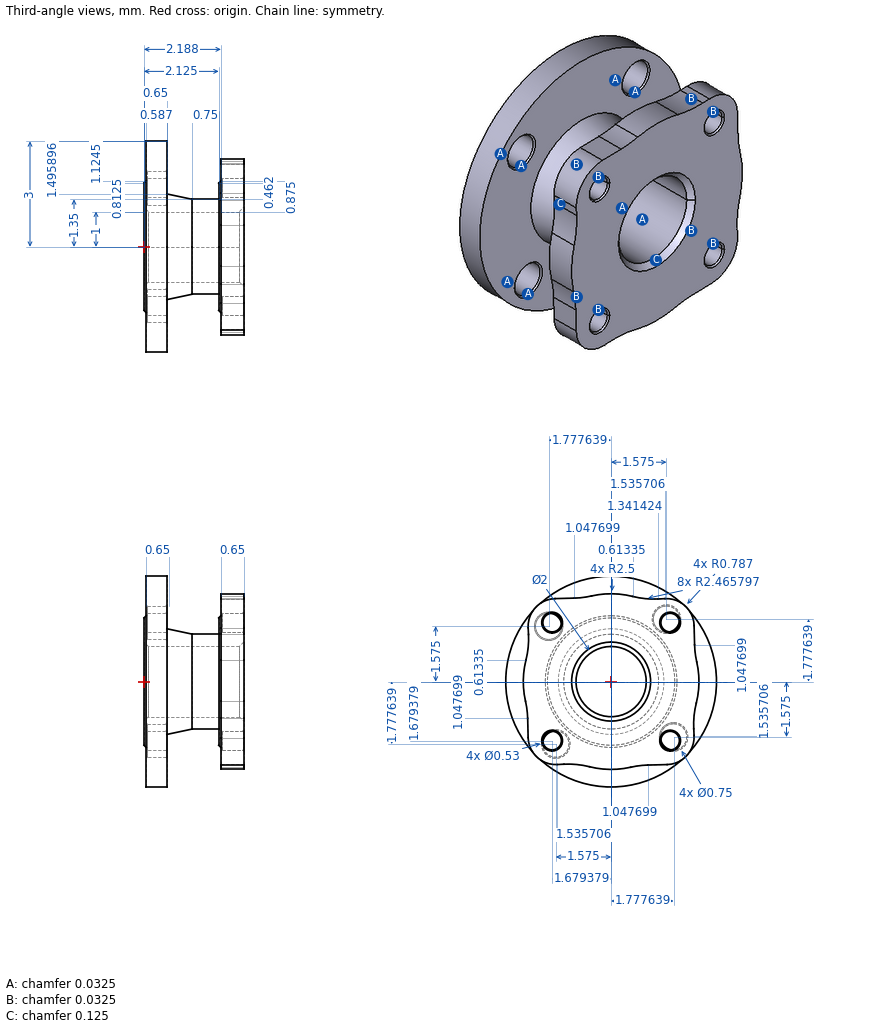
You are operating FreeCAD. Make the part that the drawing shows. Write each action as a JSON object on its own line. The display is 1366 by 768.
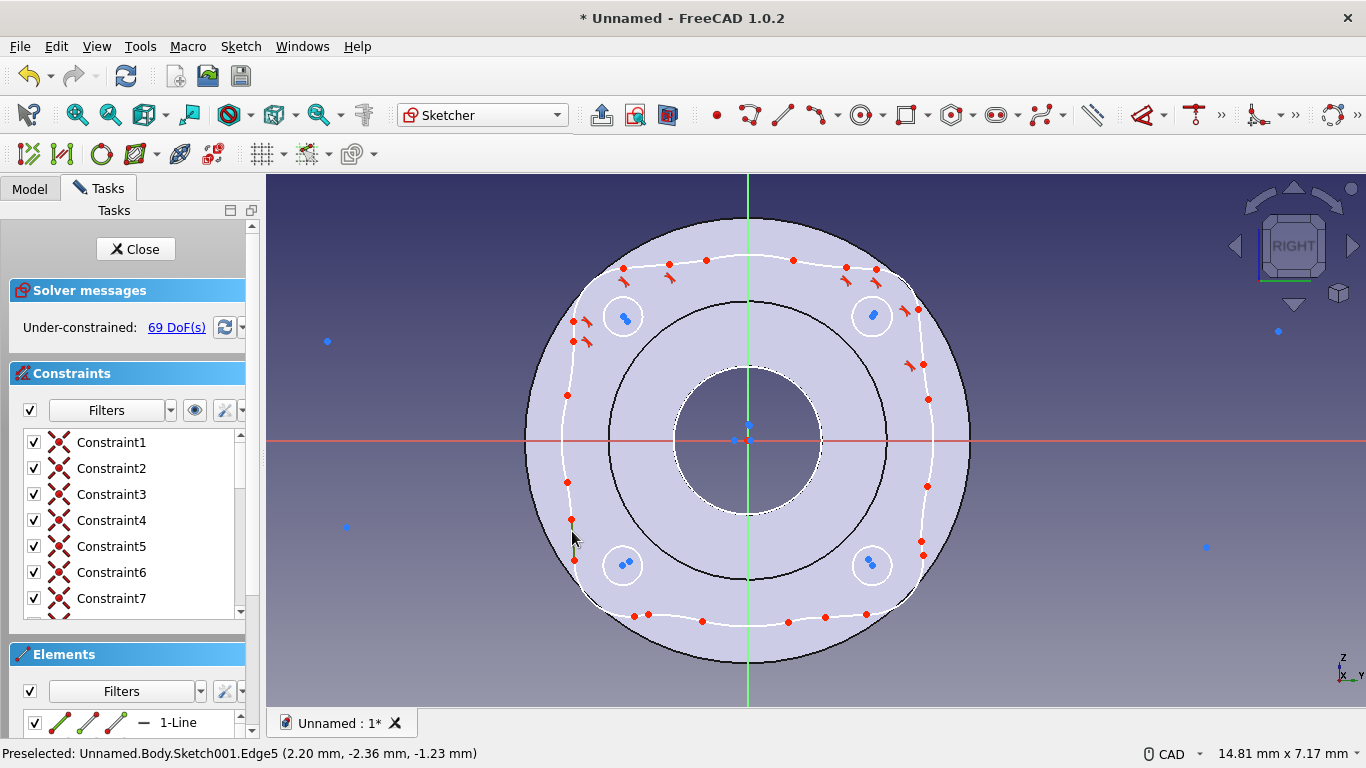
{"action": "scroll", "coordinate": [571, 508], "scroll_direction": "up", "scroll_amount": 2}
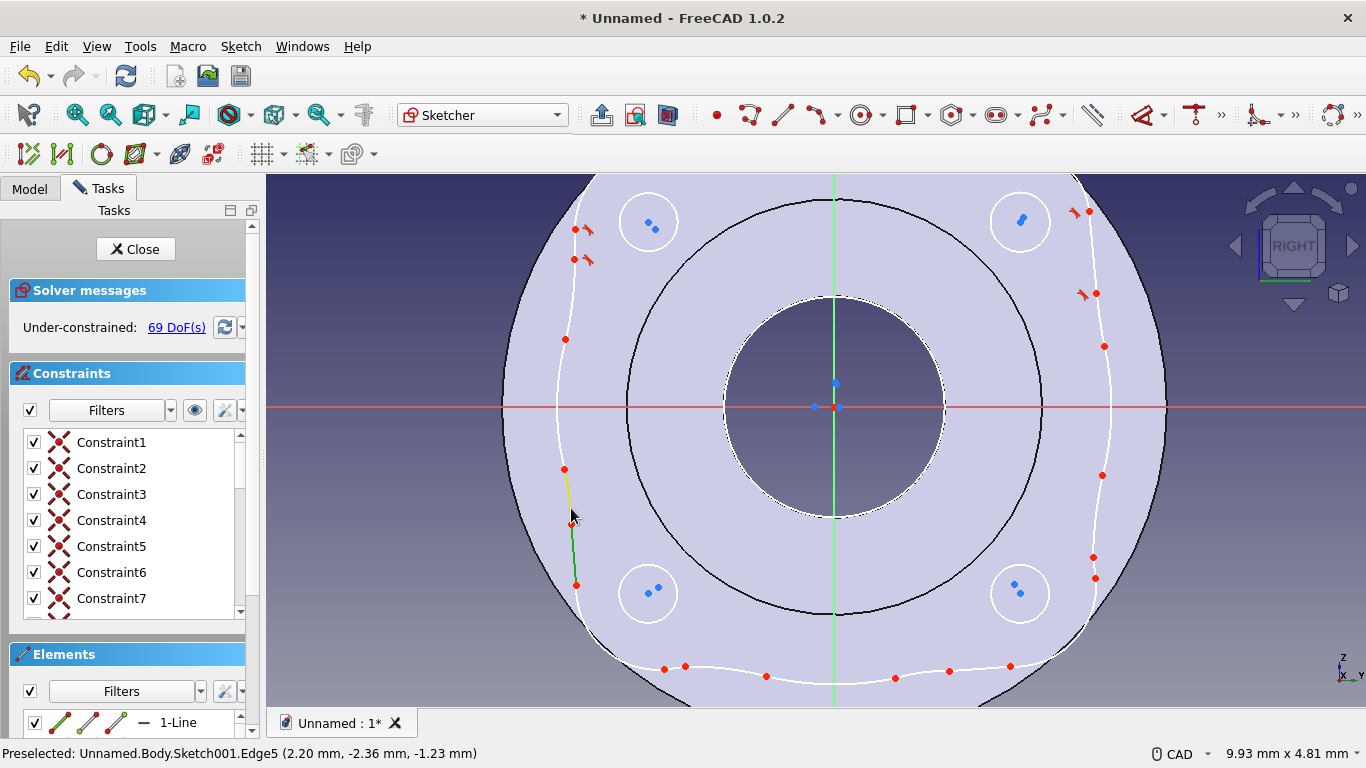
{"action": "left_click", "coordinate": [570, 508]}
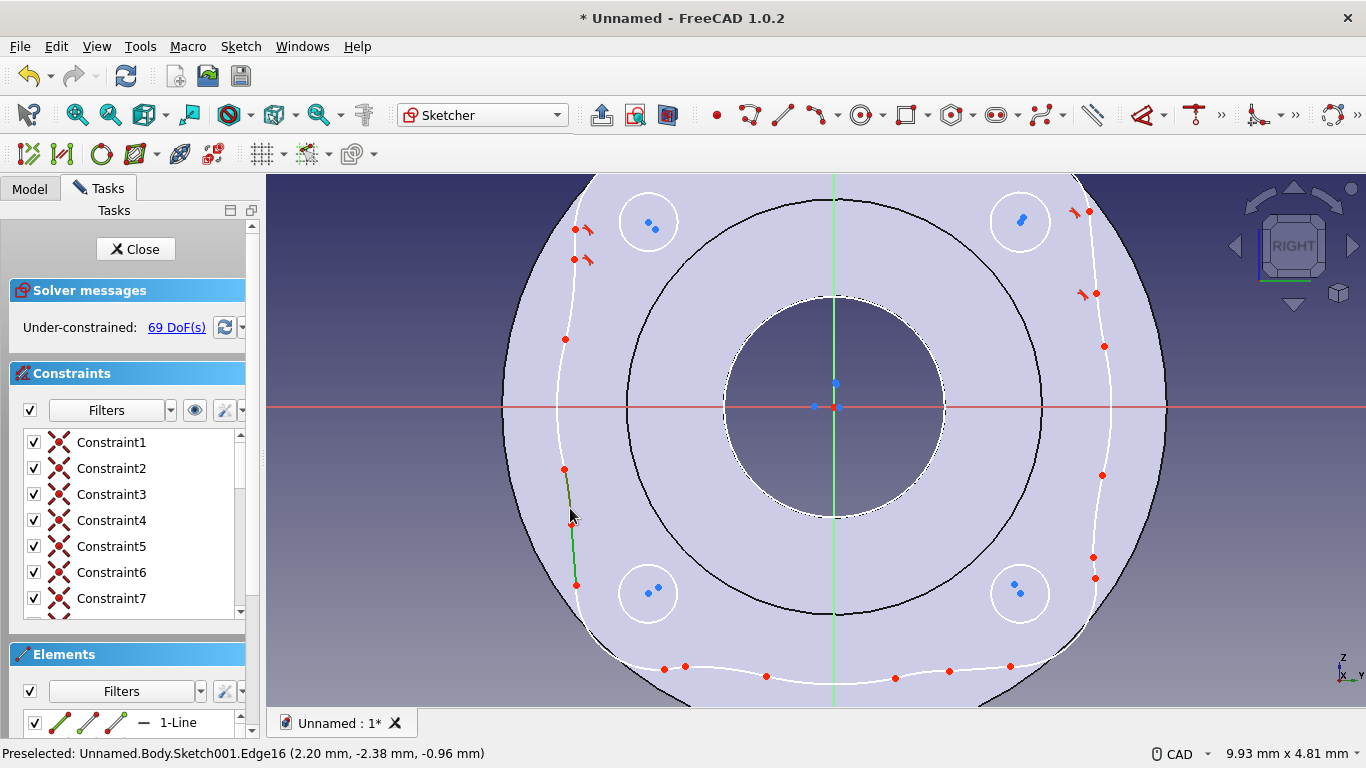
{"action": "key", "text": "t"}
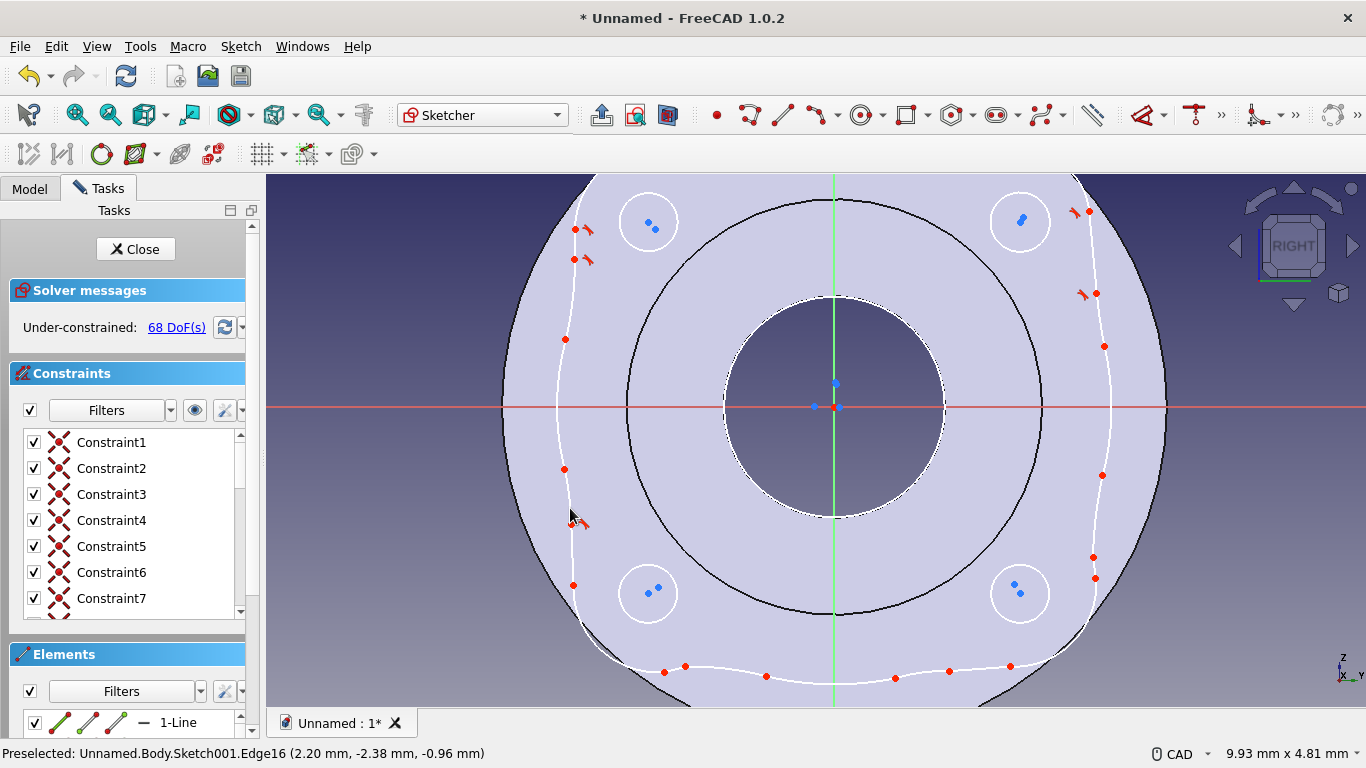
{"action": "left_click", "coordinate": [572, 543]}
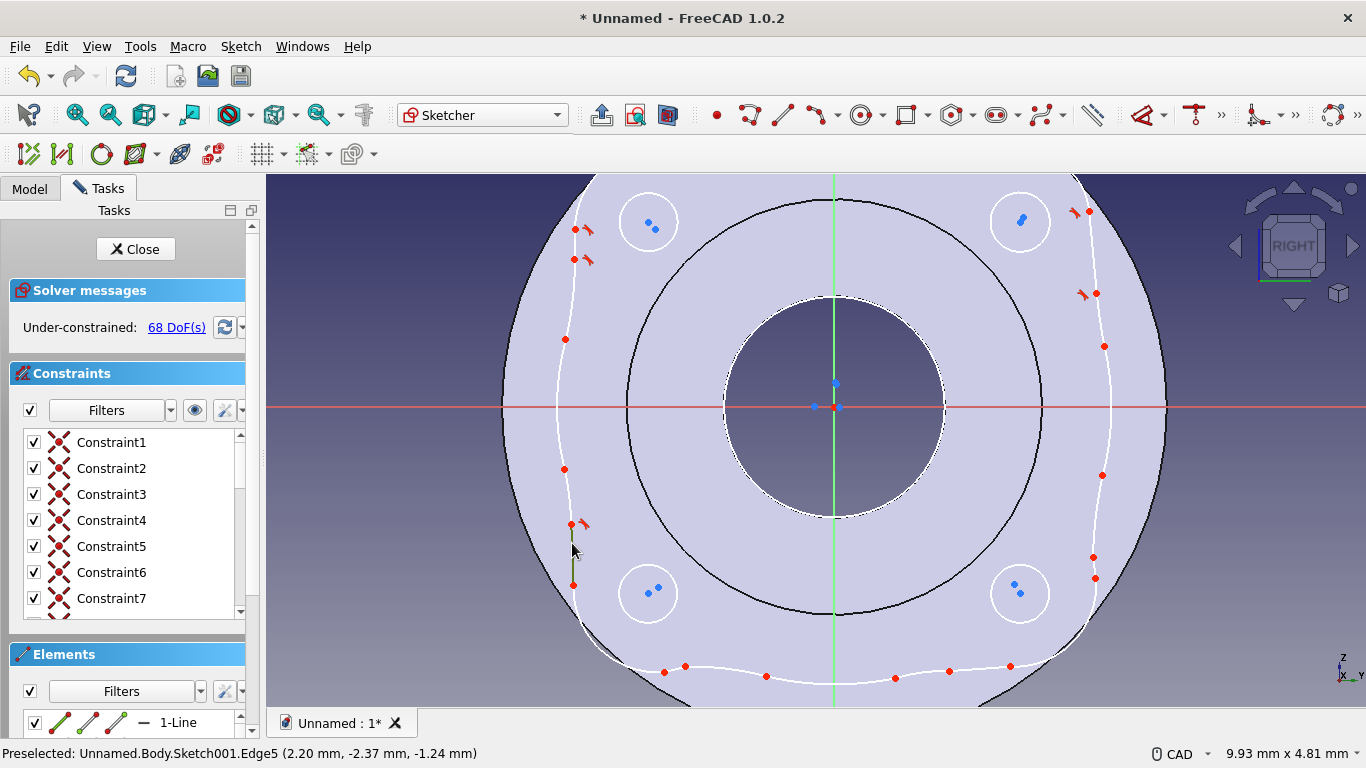
{"action": "left_click", "coordinate": [583, 626]}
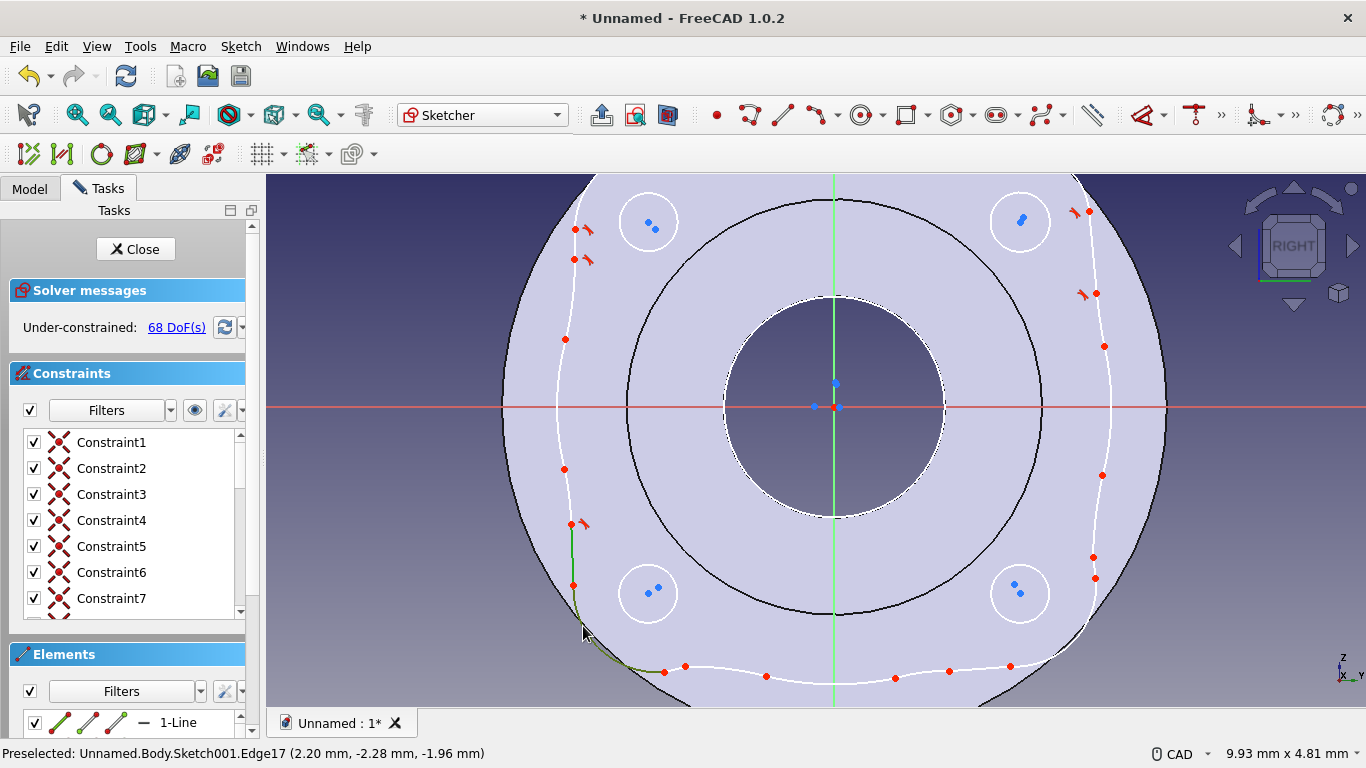
{"action": "key", "text": "t"}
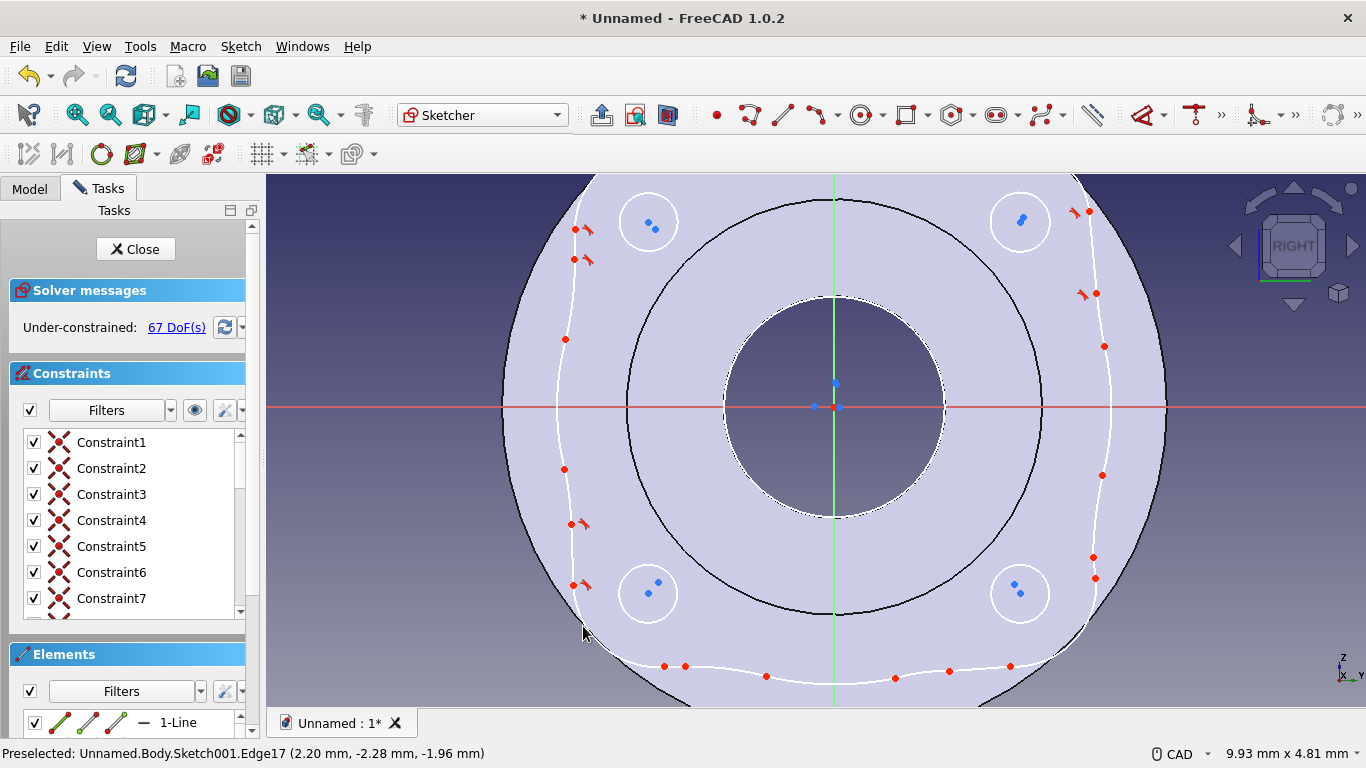
{"action": "scroll", "coordinate": [675, 667], "scroll_direction": "up", "scroll_amount": 2}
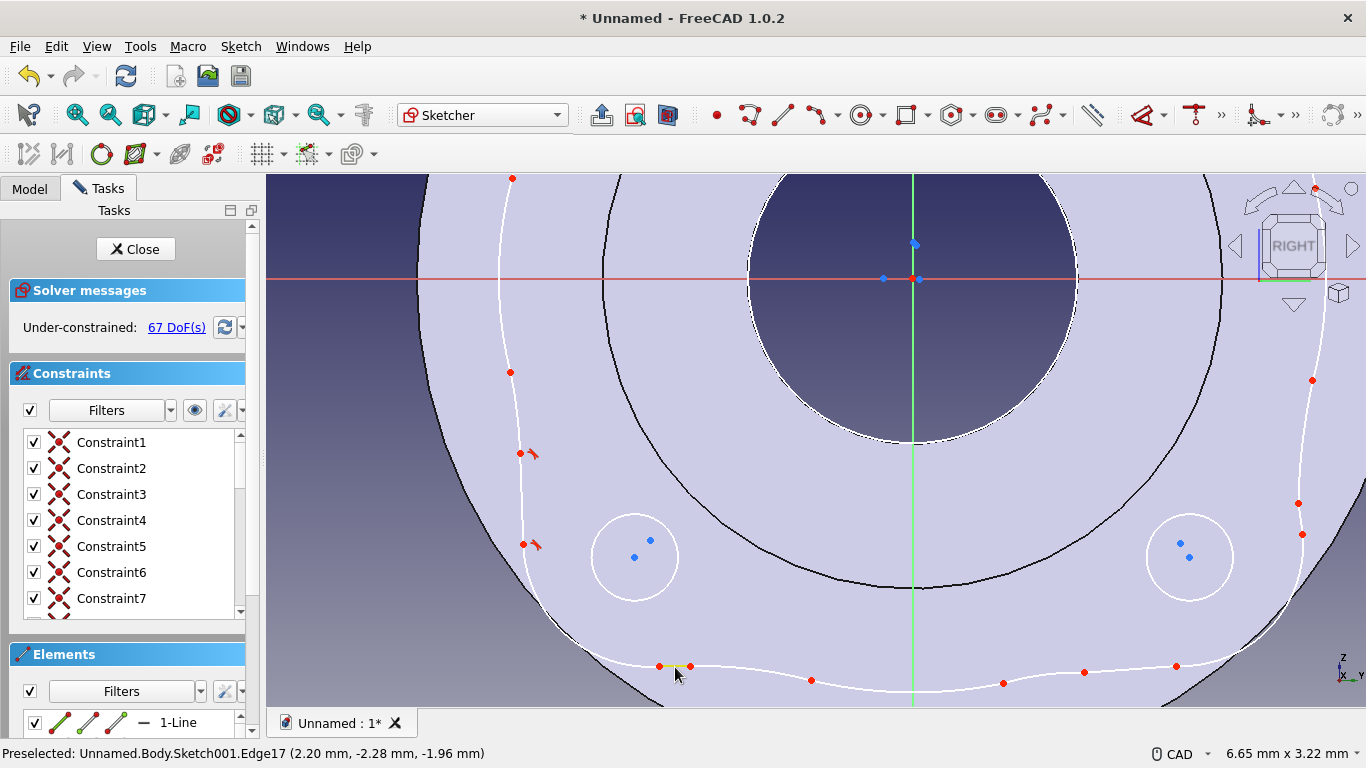
{"action": "left_click", "coordinate": [675, 666]}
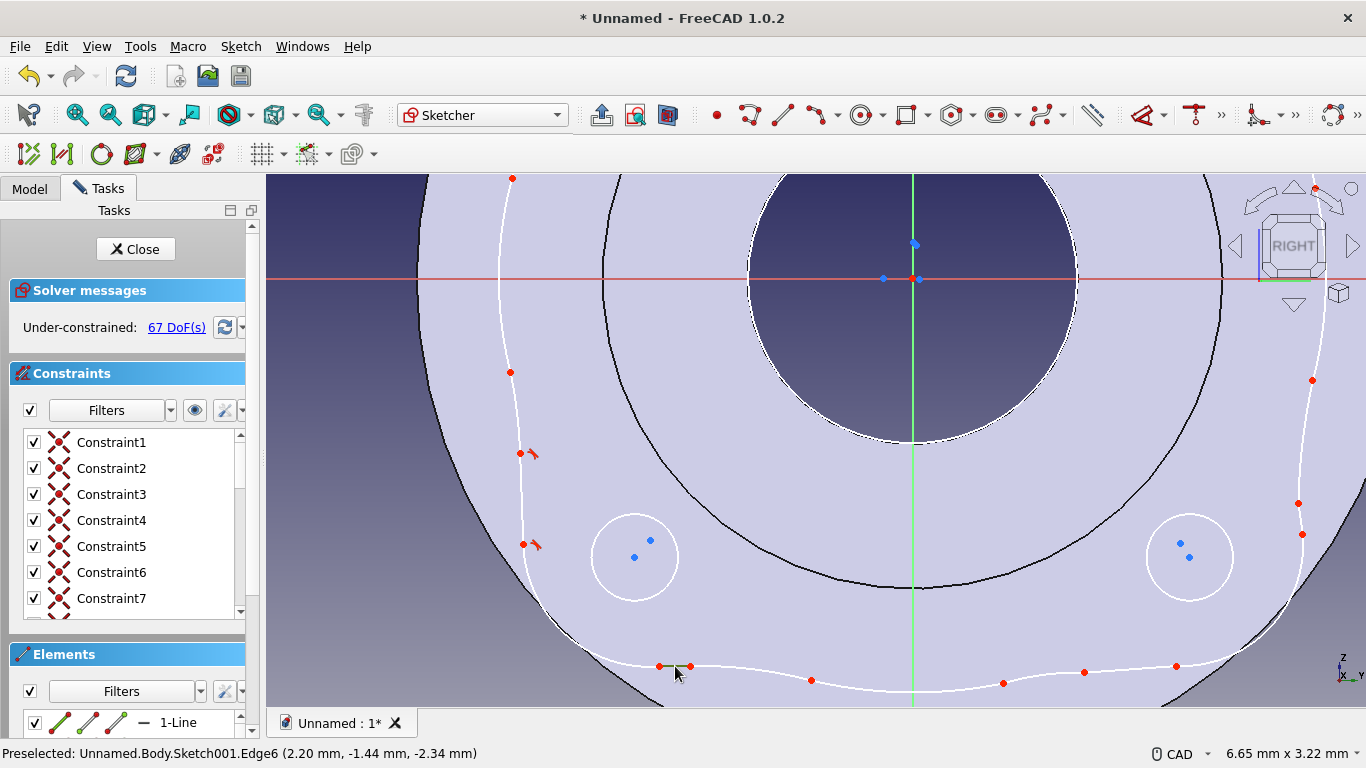
{"action": "left_click", "coordinate": [540, 603]}